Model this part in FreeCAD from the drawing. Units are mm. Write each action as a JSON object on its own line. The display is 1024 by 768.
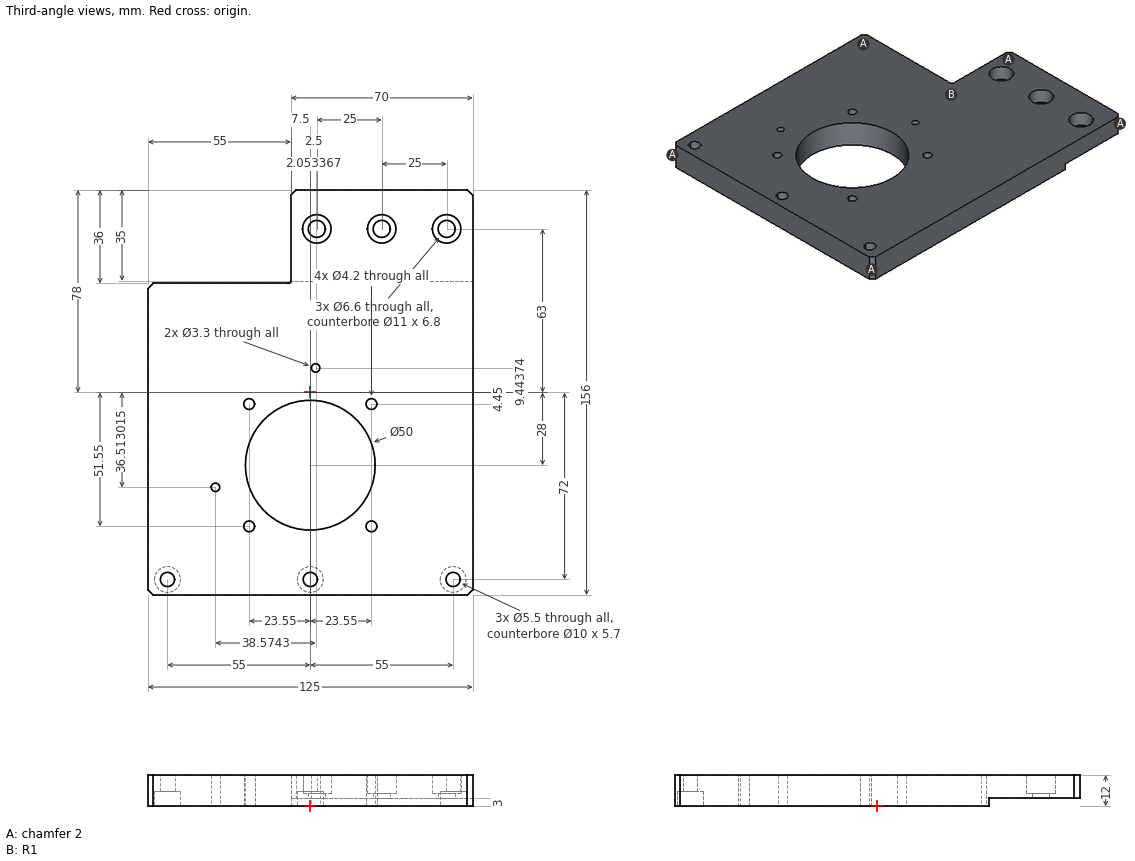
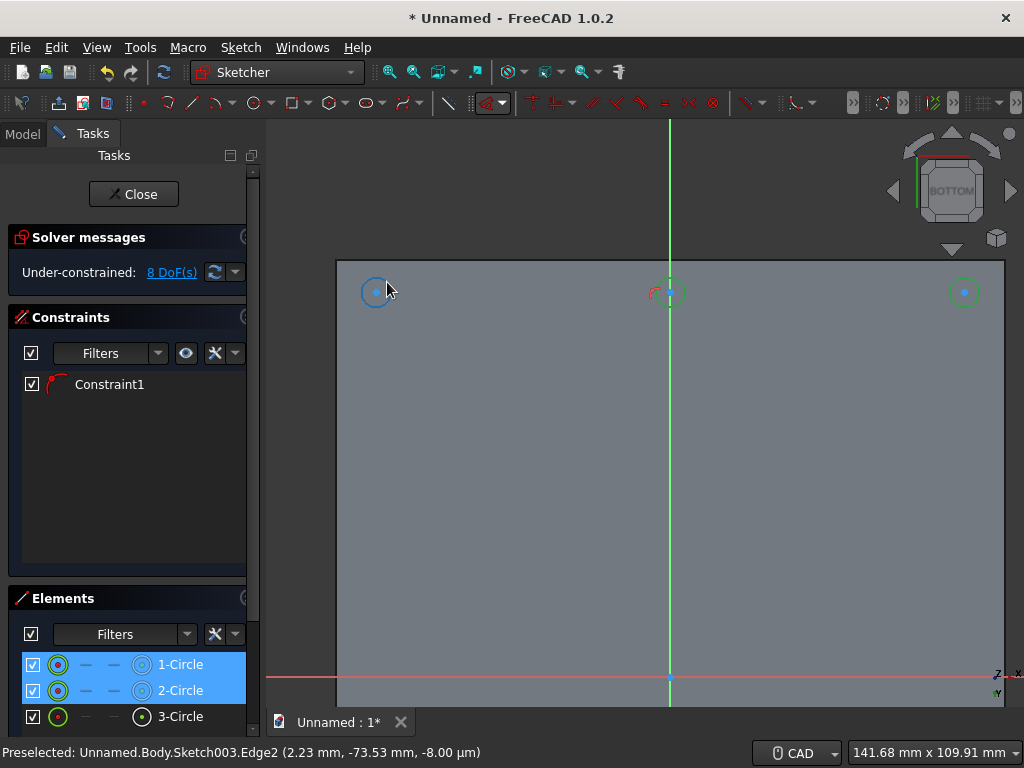
{"action": "left_click", "coordinate": [387, 282]}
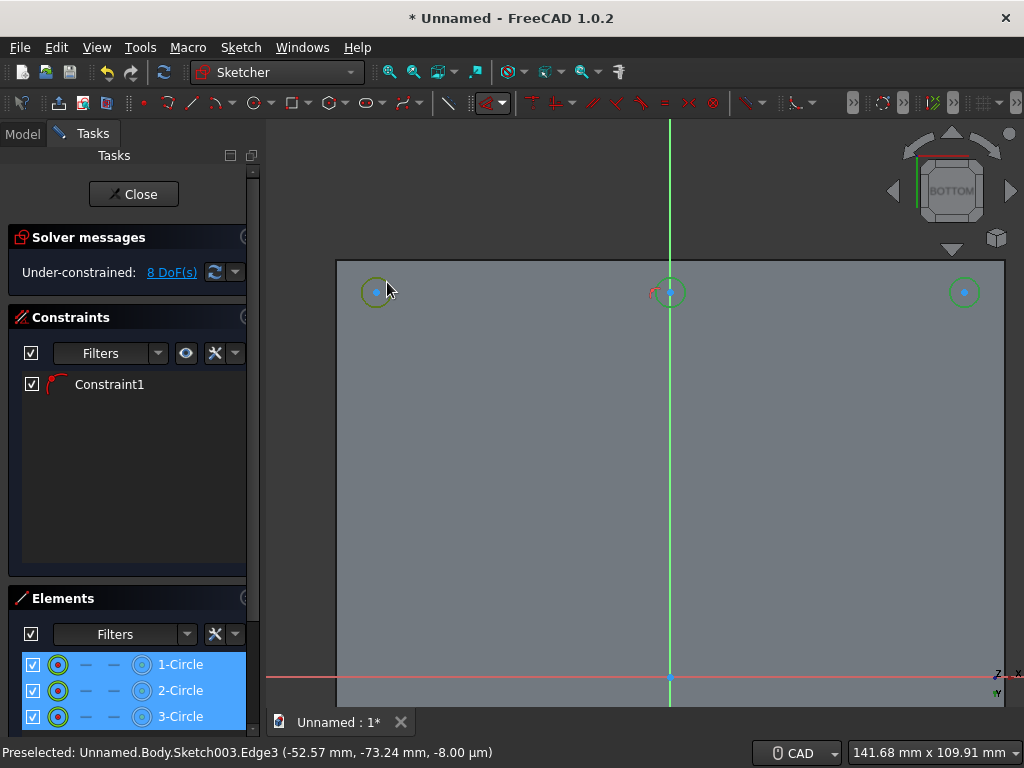
{"action": "left_click", "coordinate": [666, 104]}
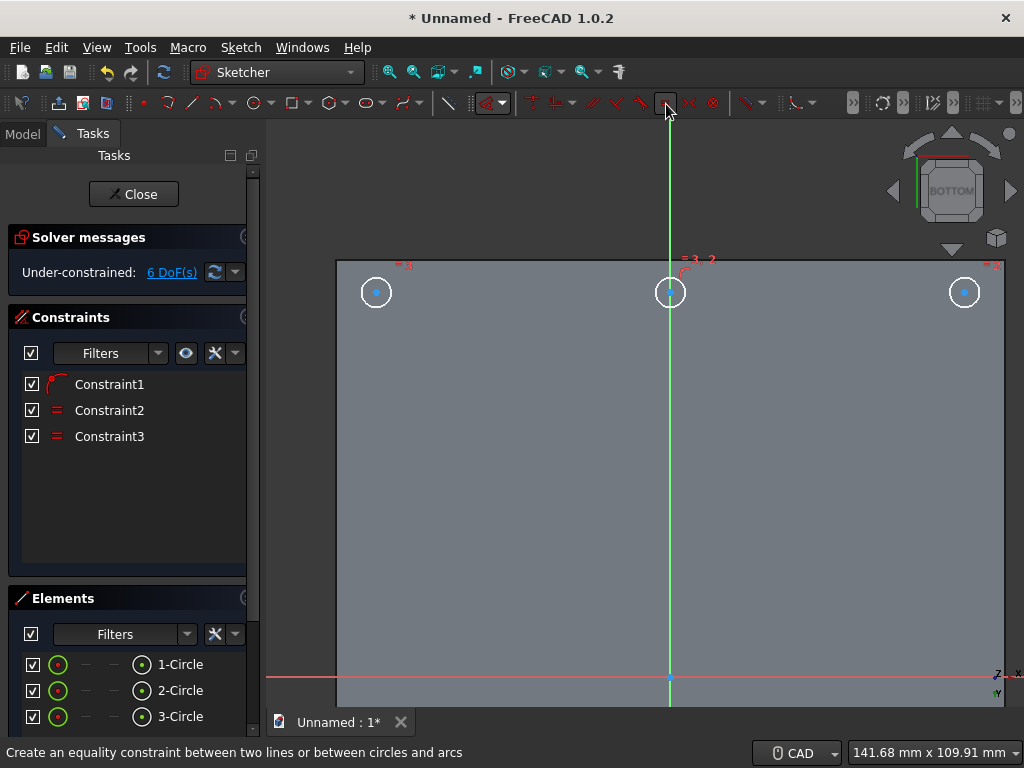
{"action": "scroll", "coordinate": [385, 282], "scroll_direction": "down", "scroll_amount": 2}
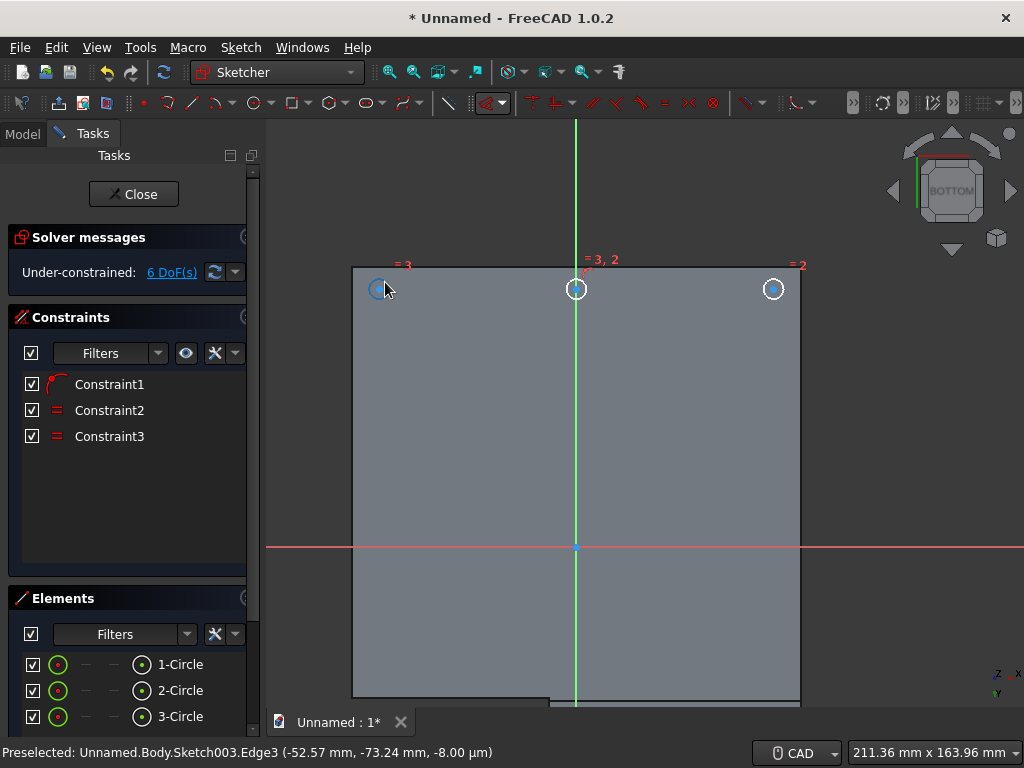
{"action": "left_click", "coordinate": [774, 289]}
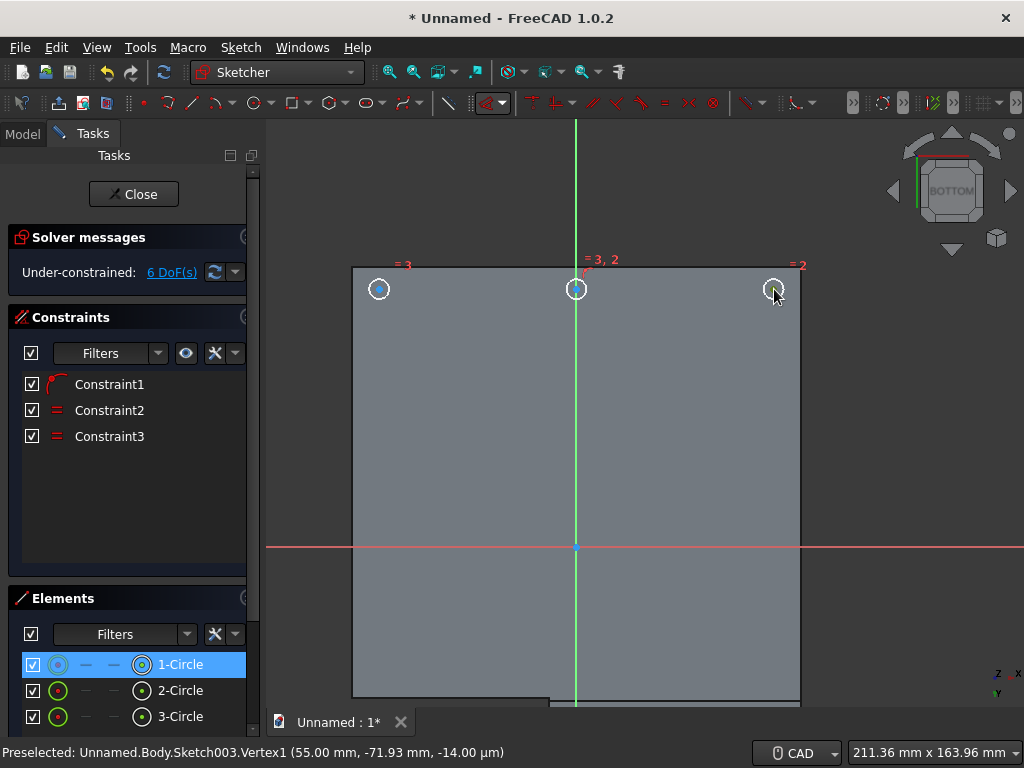
{"action": "left_click", "coordinate": [576, 289]}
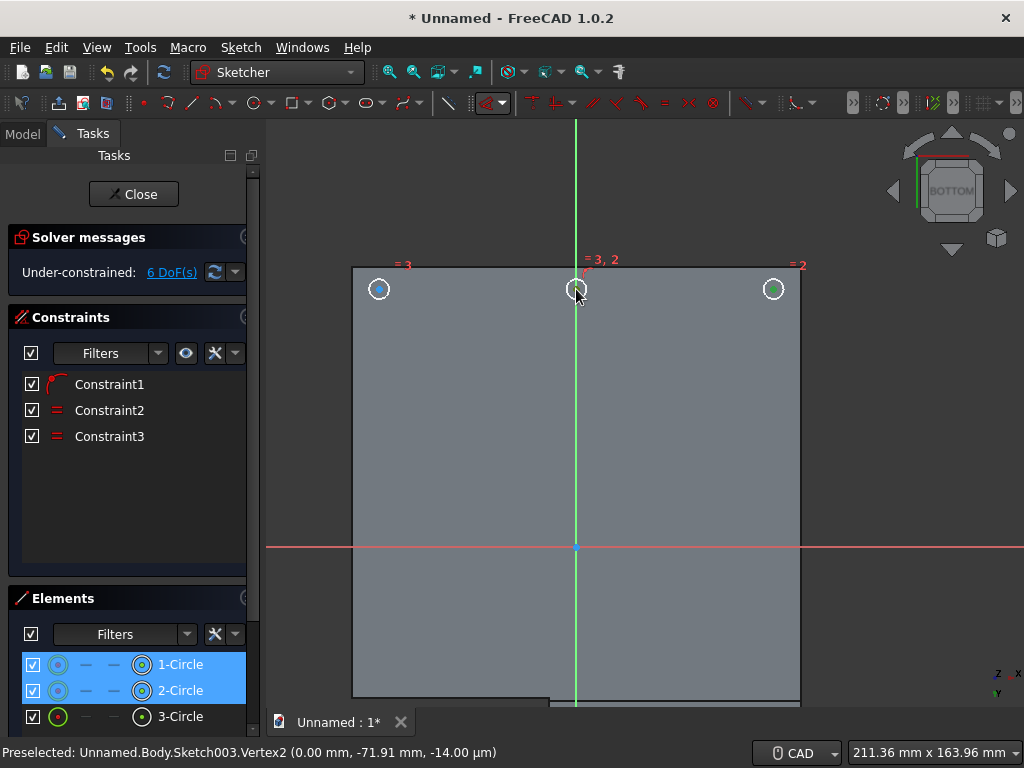
{"action": "left_click", "coordinate": [574, 104]}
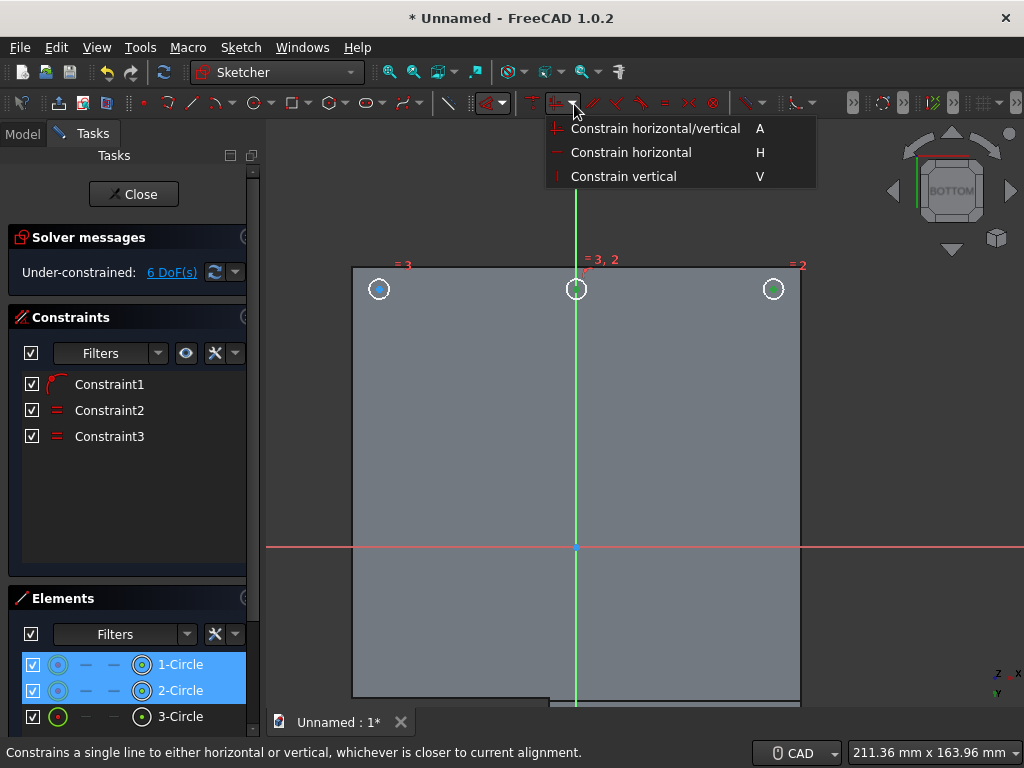
{"action": "left_click", "coordinate": [681, 152]}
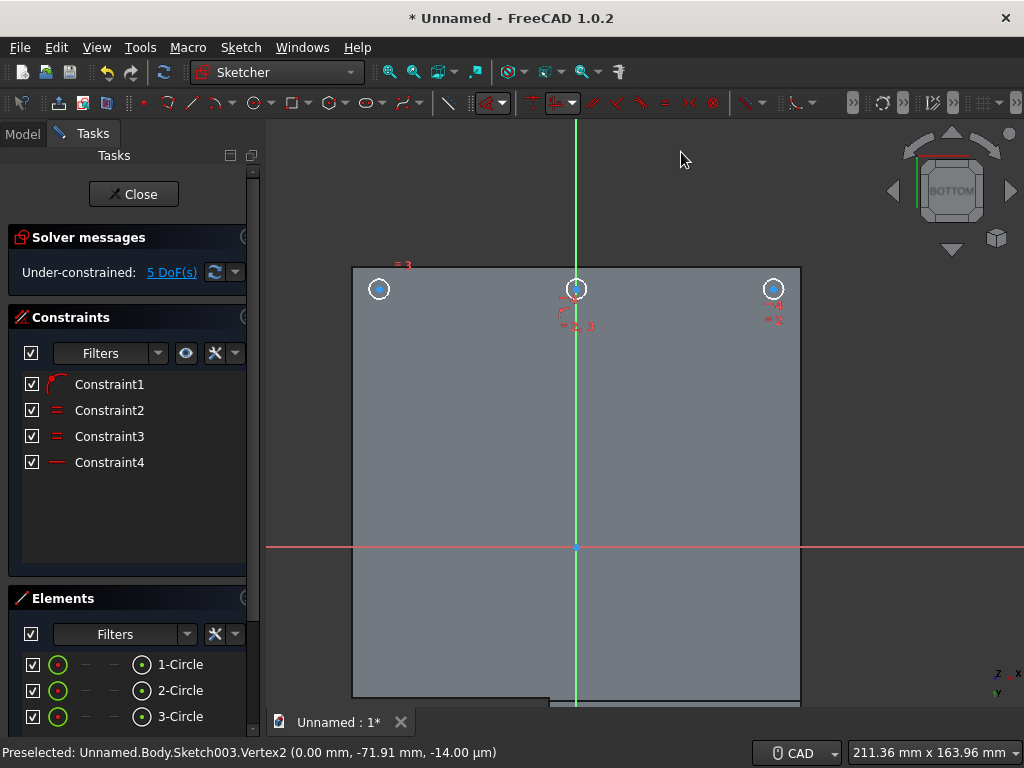
{"action": "left_click", "coordinate": [576, 289]}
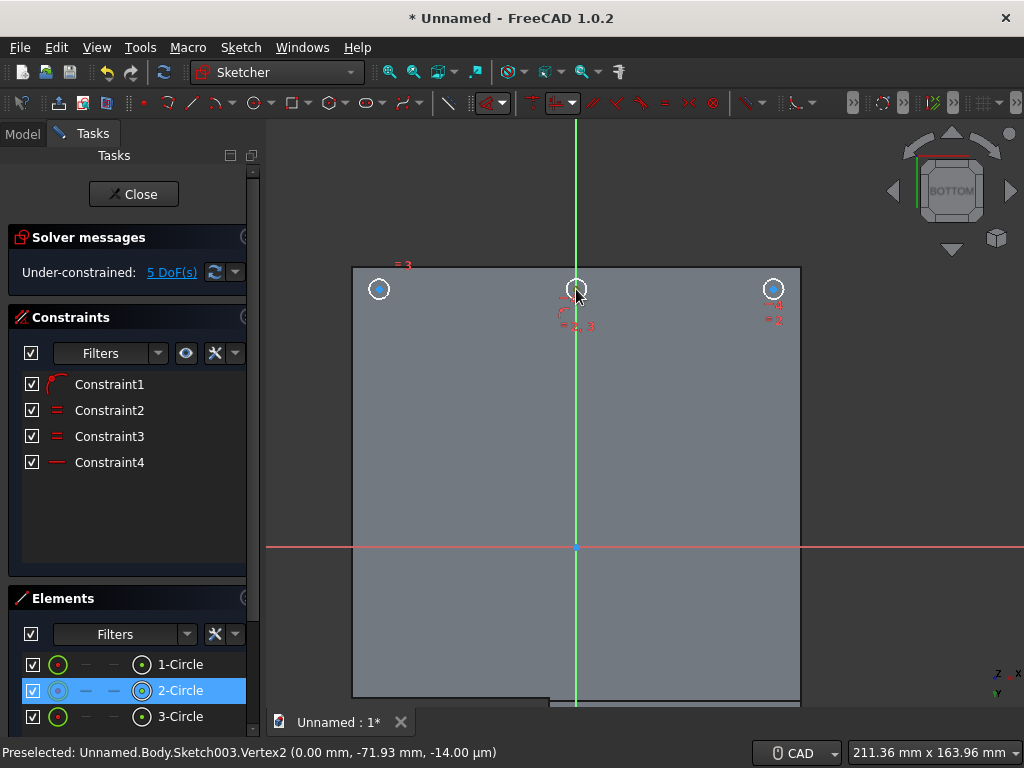
{"action": "left_click", "coordinate": [379, 289]}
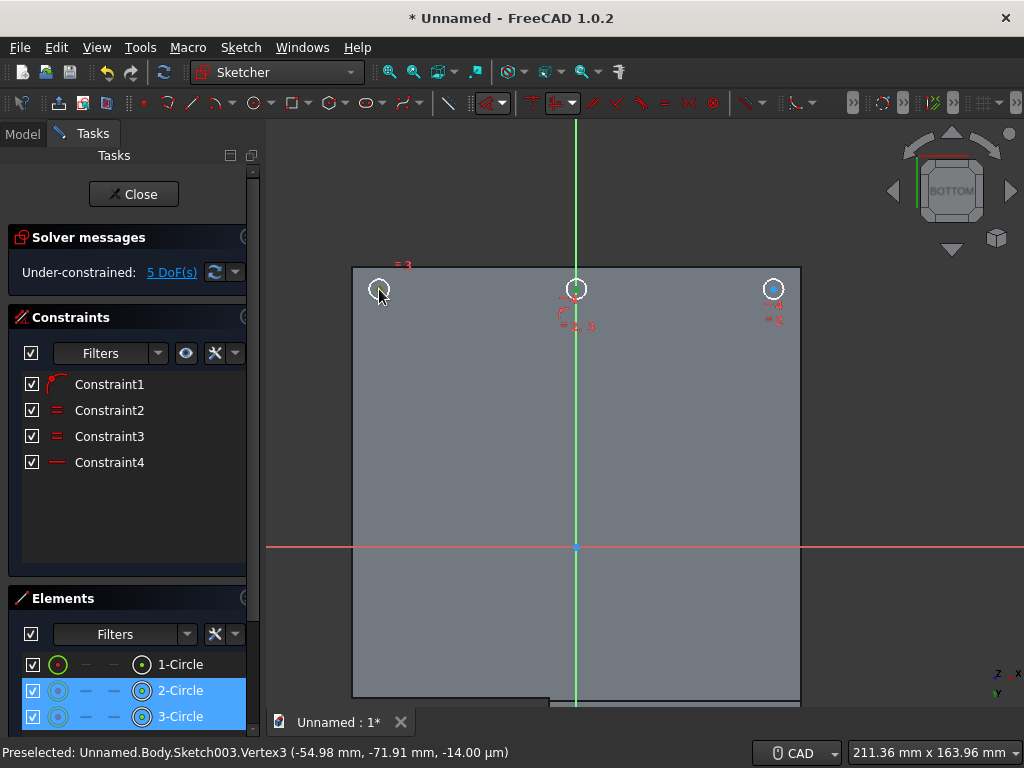
{"action": "left_click", "coordinate": [574, 104]}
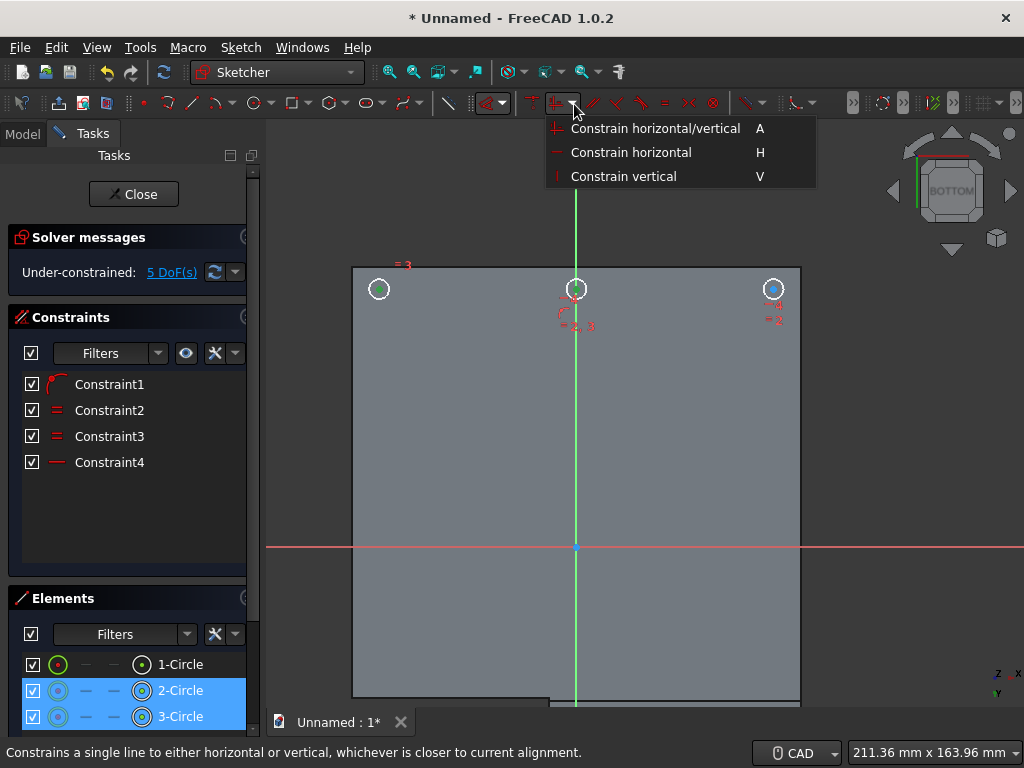
{"action": "left_click", "coordinate": [681, 152]}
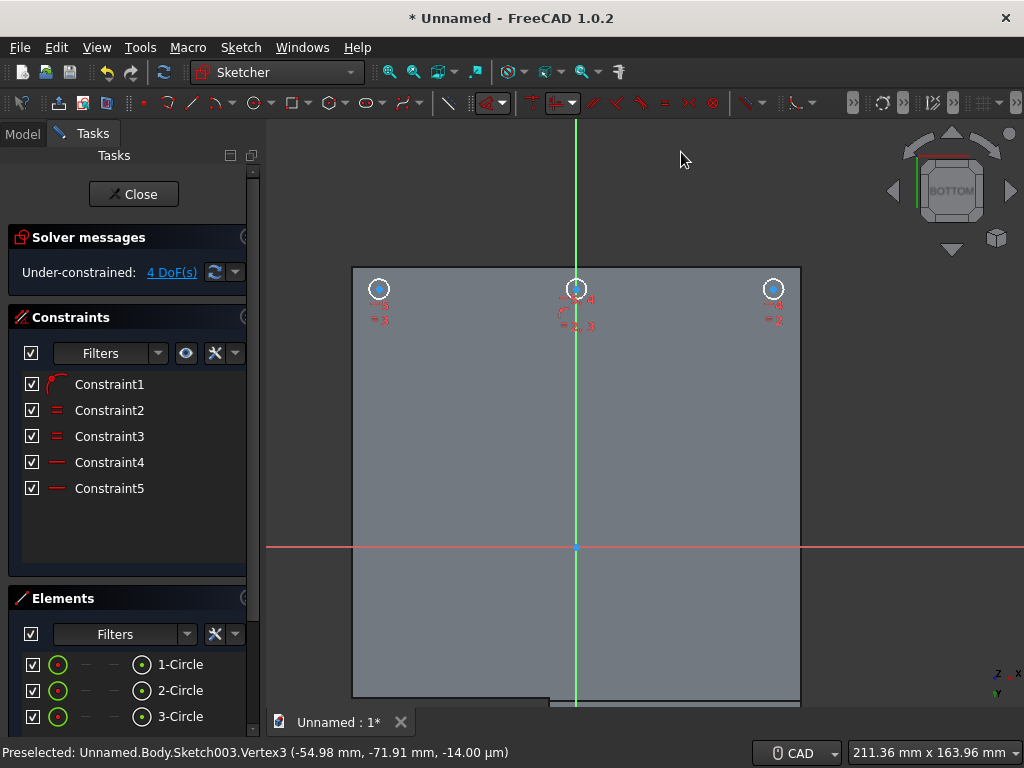
{"action": "scroll", "coordinate": [781, 282], "scroll_direction": "up", "scroll_amount": 4}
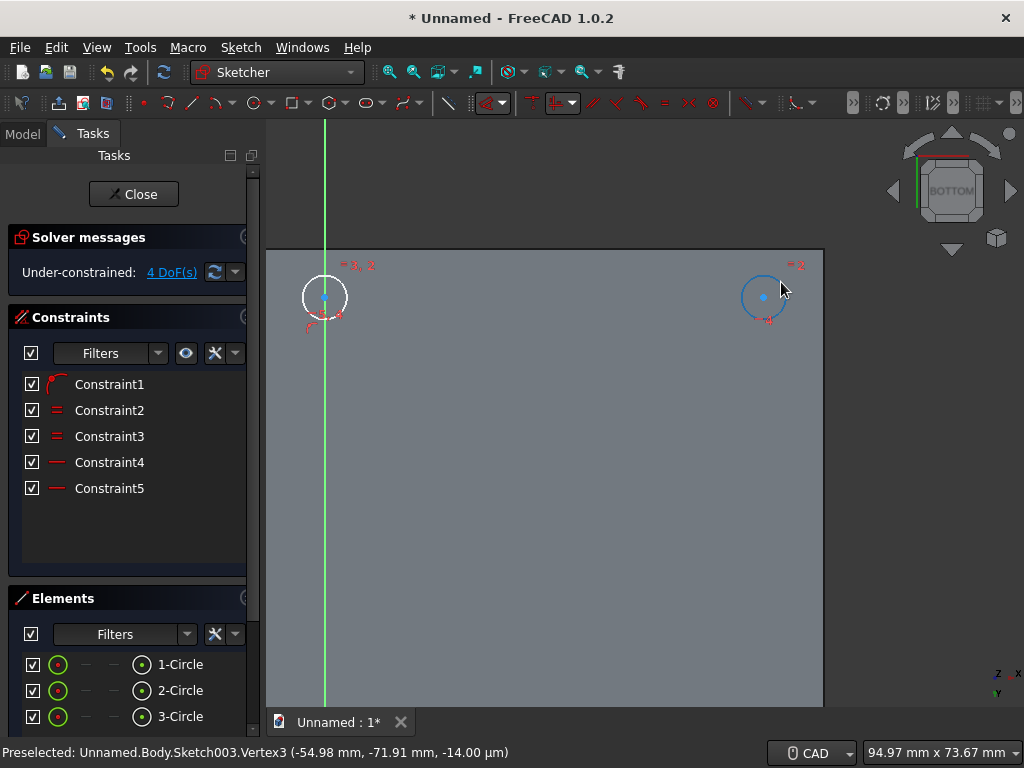
{"action": "left_click", "coordinate": [779, 282]}